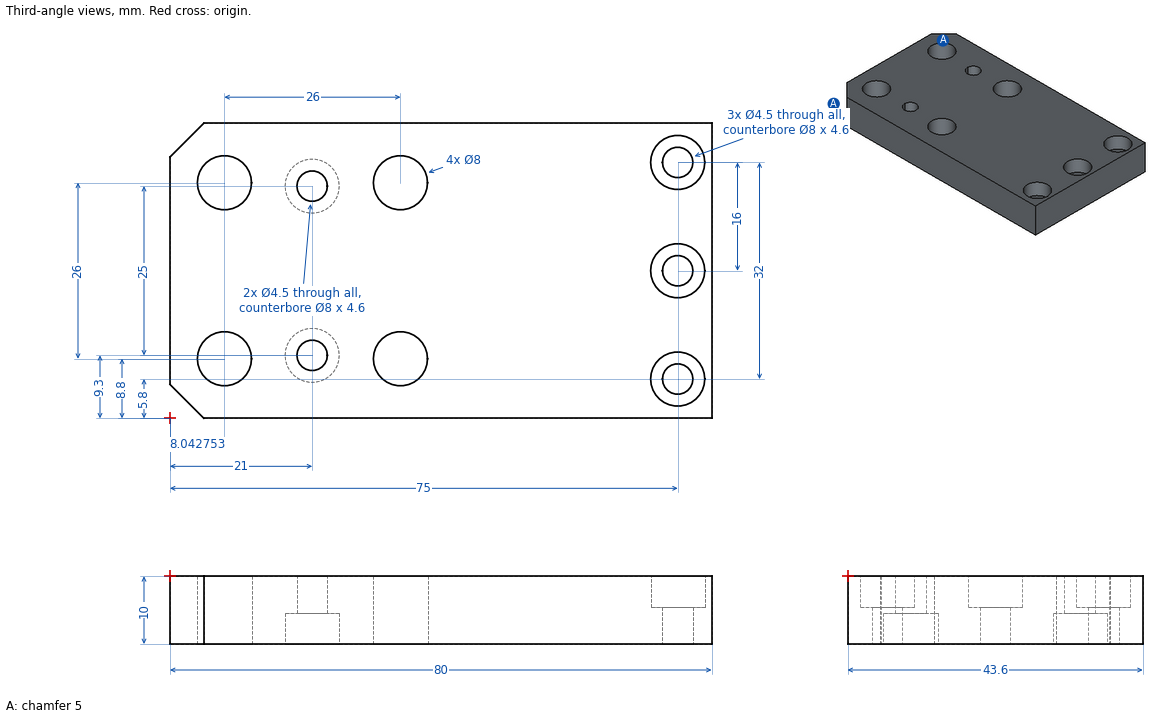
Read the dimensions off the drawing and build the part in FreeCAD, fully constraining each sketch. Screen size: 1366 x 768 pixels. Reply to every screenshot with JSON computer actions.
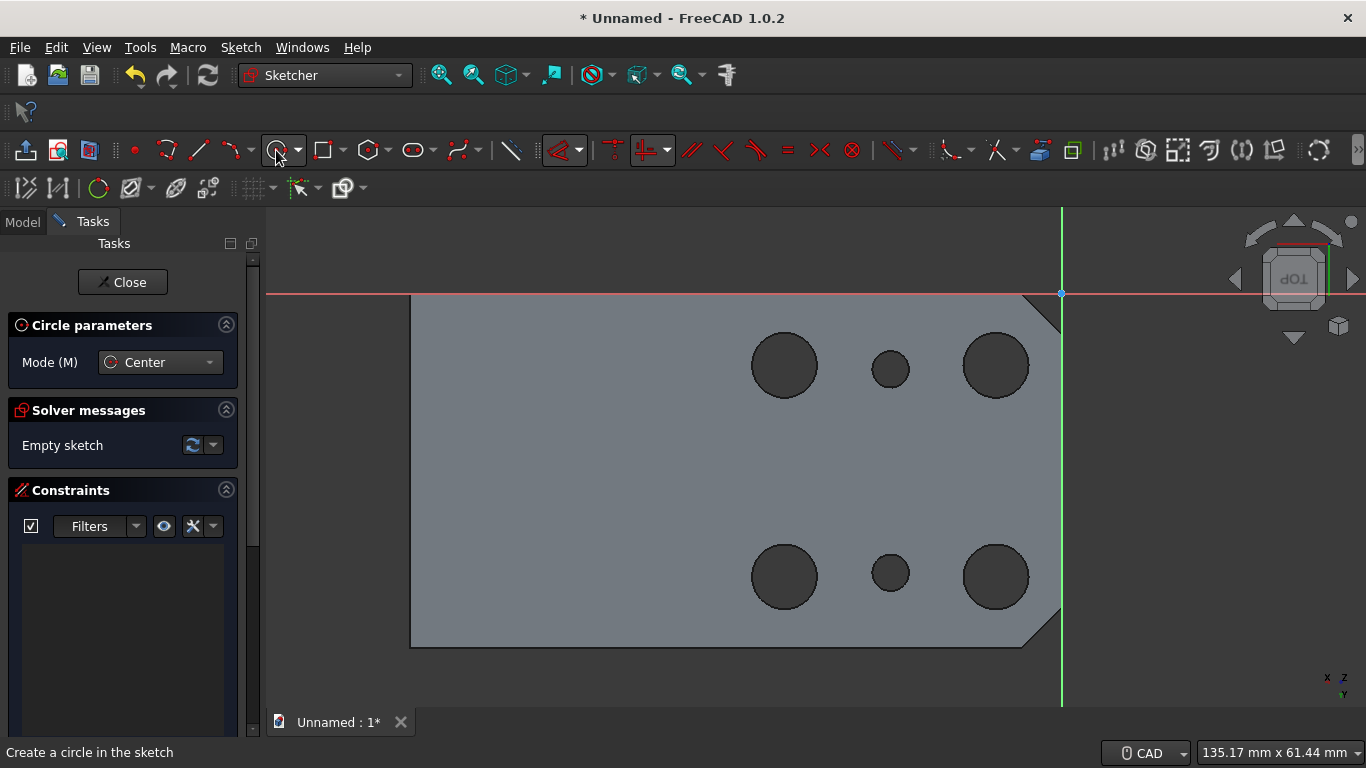
{"action": "scroll", "coordinate": [451, 601], "scroll_direction": "up", "scroll_amount": 2}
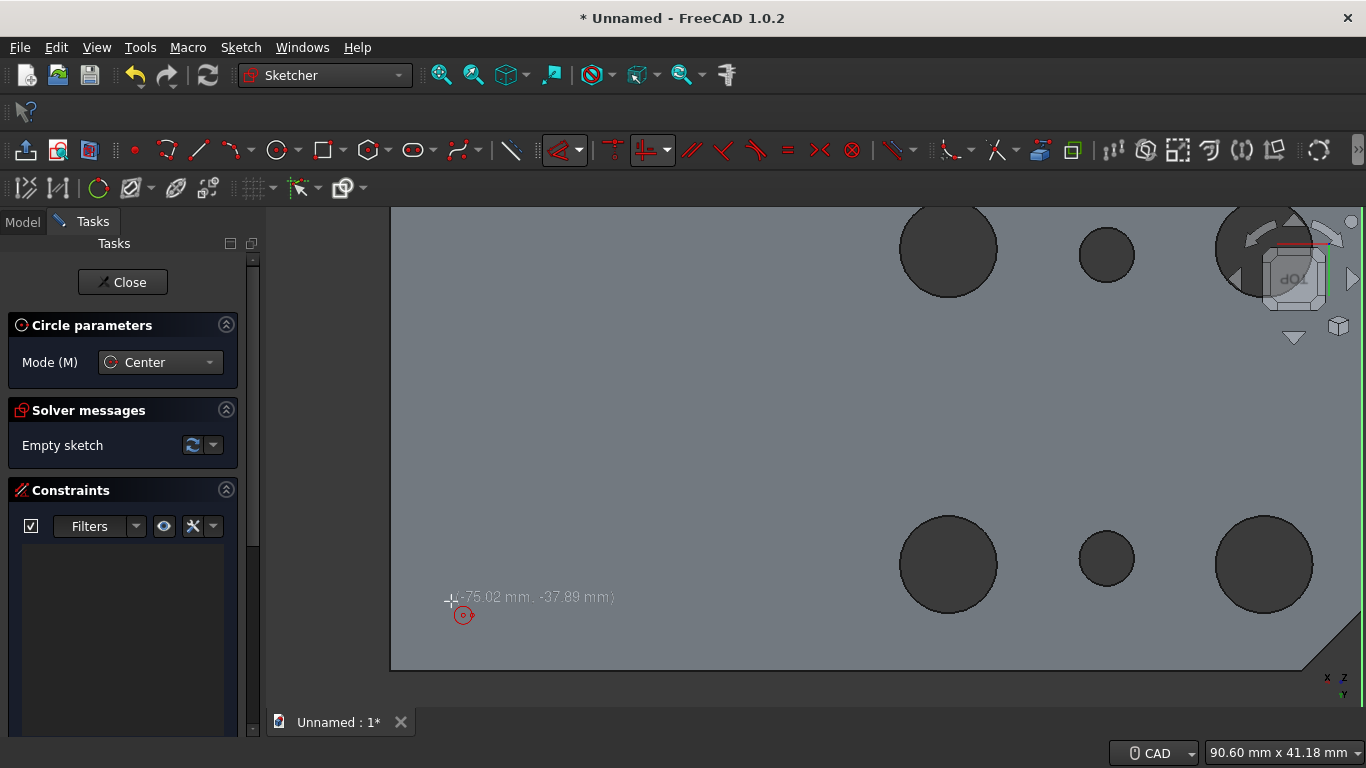
{"action": "left_click", "coordinate": [451, 601]}
{"action": "left_click", "coordinate": [470, 582]}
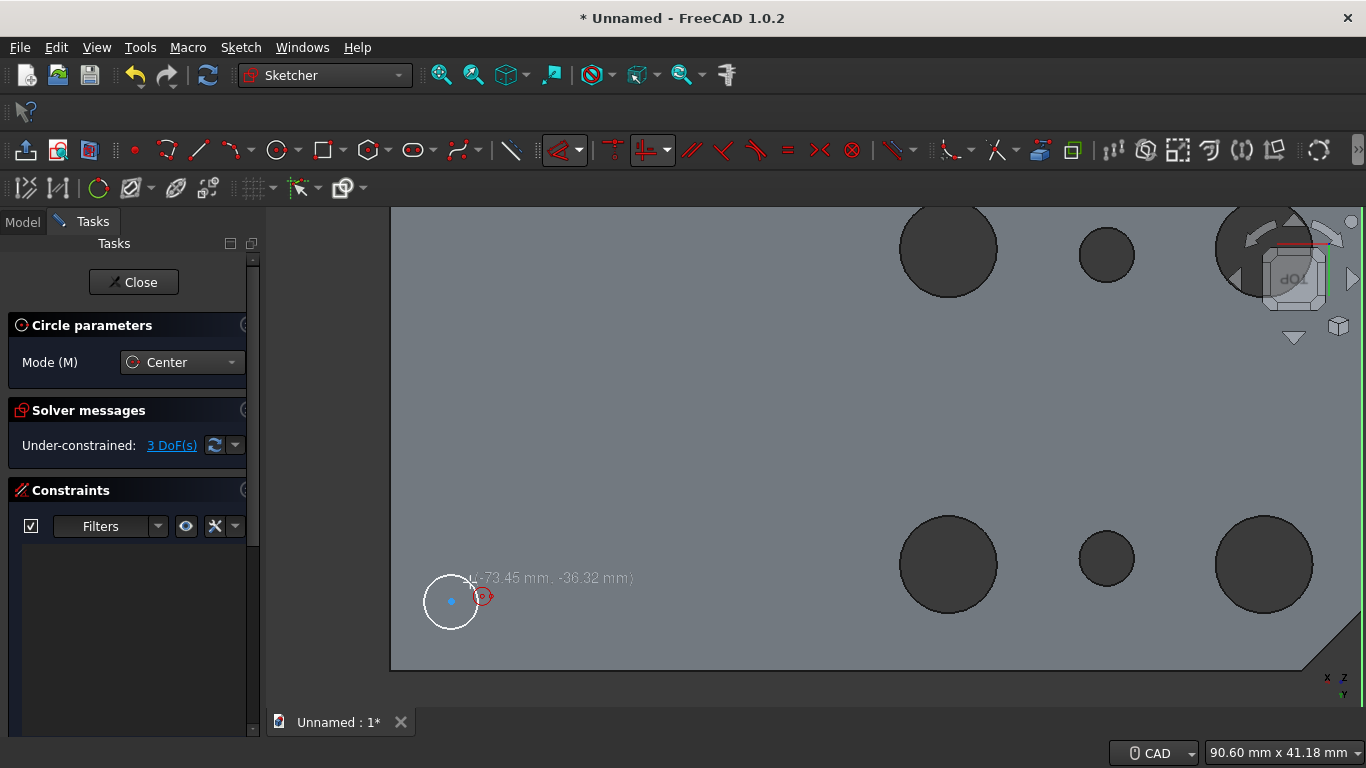
{"action": "scroll", "coordinate": [452, 603], "scroll_direction": "down", "scroll_amount": 2}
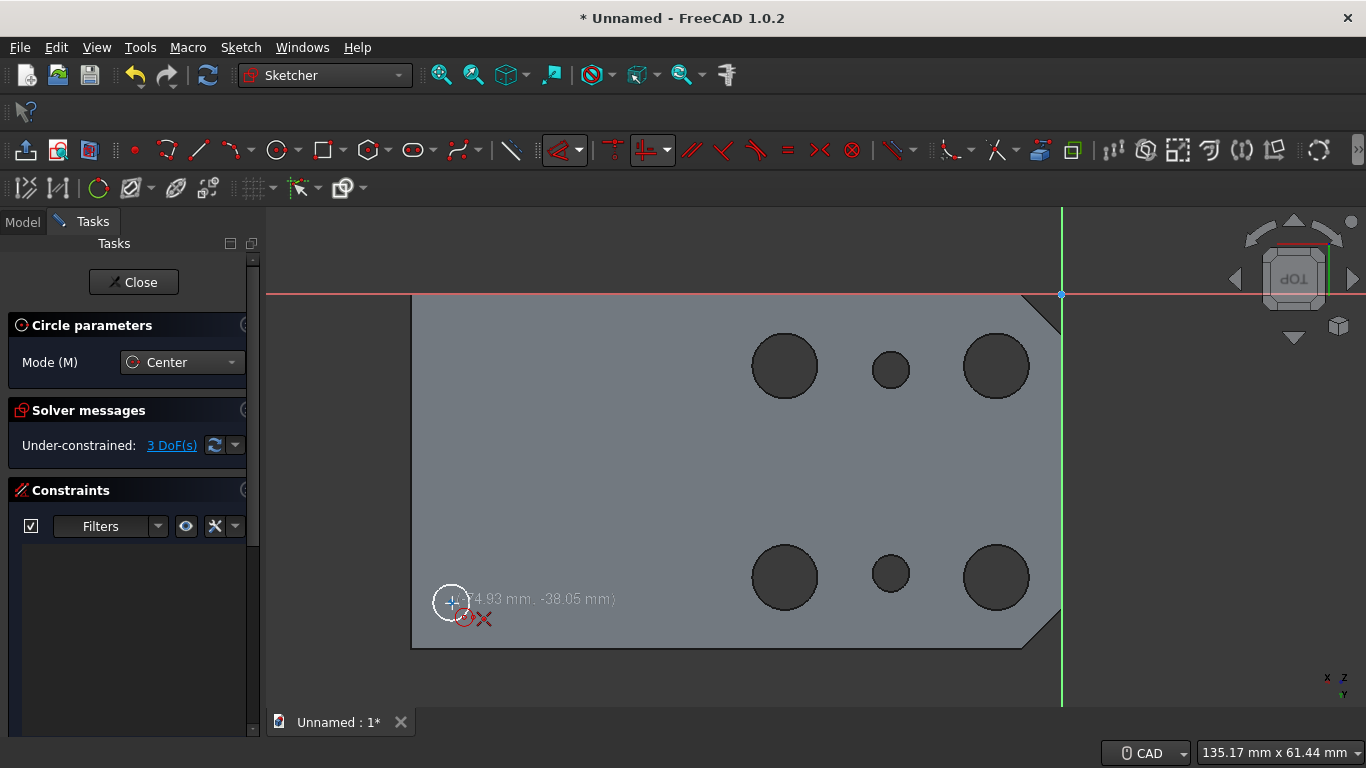
{"action": "scroll", "coordinate": [452, 341], "scroll_direction": "up", "scroll_amount": 2}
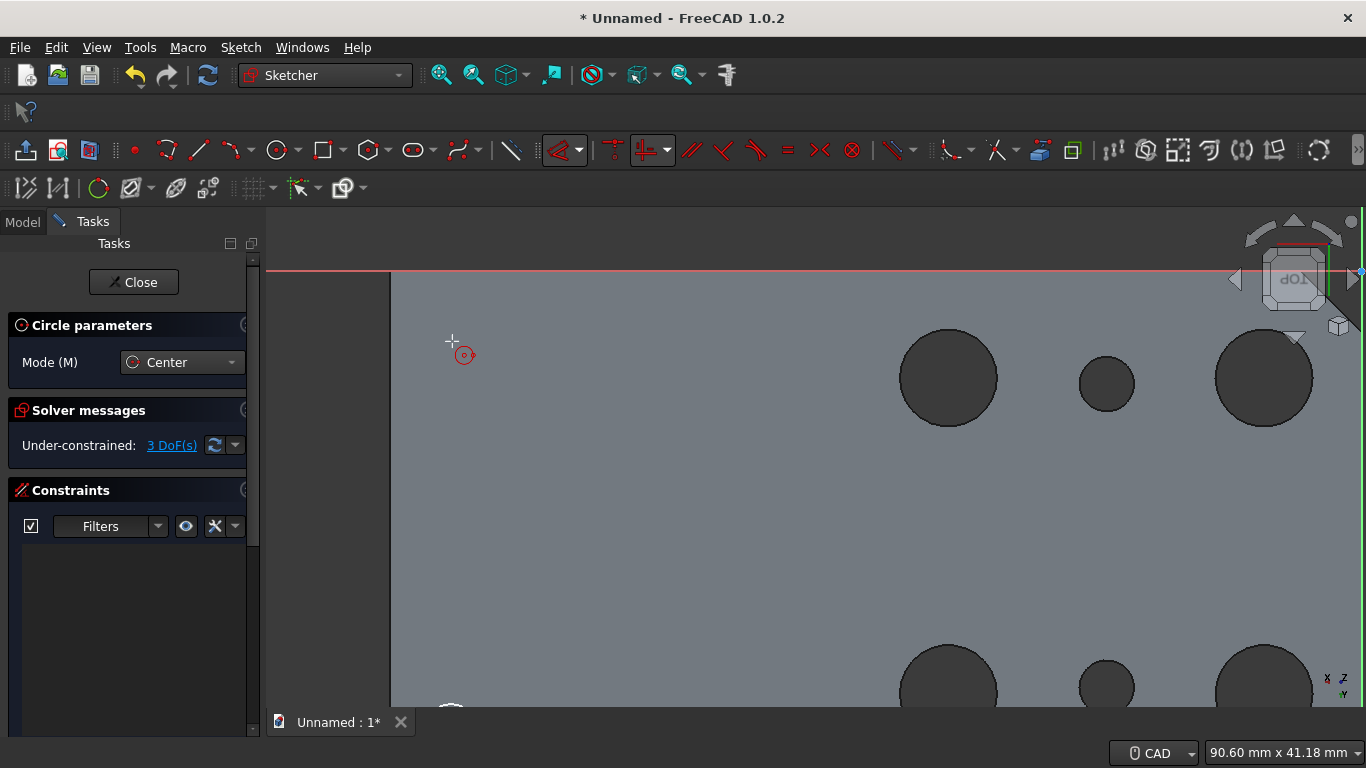
{"action": "left_click", "coordinate": [451, 342]}
{"action": "left_click", "coordinate": [470, 322]}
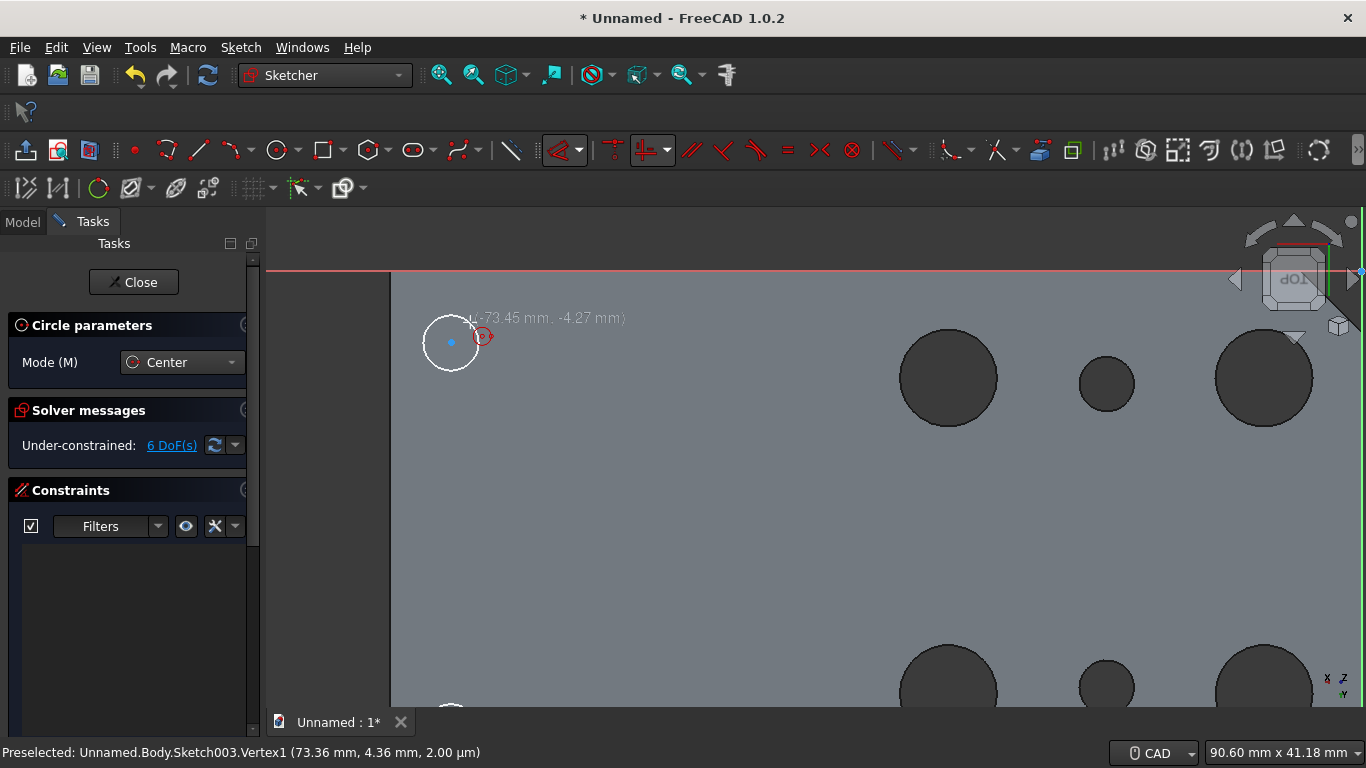
{"action": "left_click", "coordinate": [451, 536]}
{"action": "left_click", "coordinate": [470, 517]}
{"action": "key", "text": "Escape"}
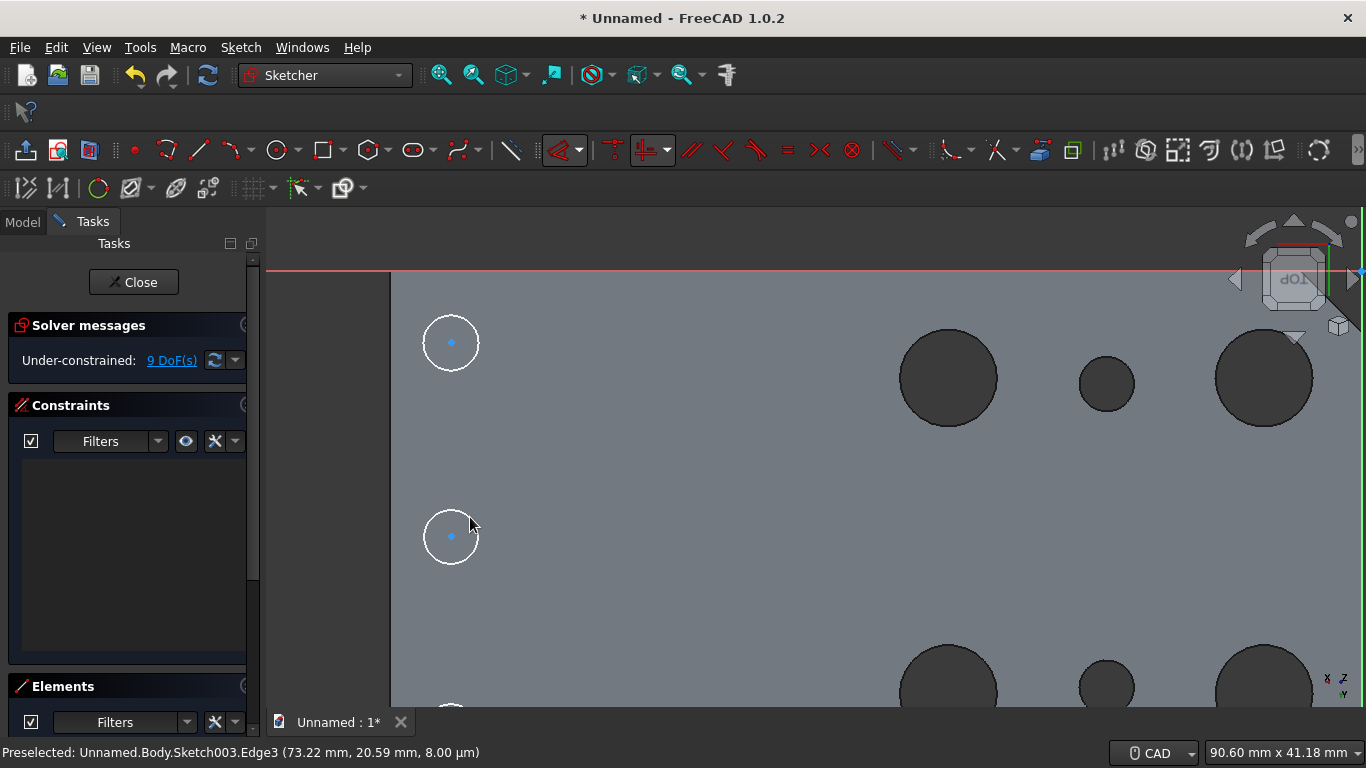
{"action": "scroll", "coordinate": [452, 340], "scroll_direction": "down", "scroll_amount": 2}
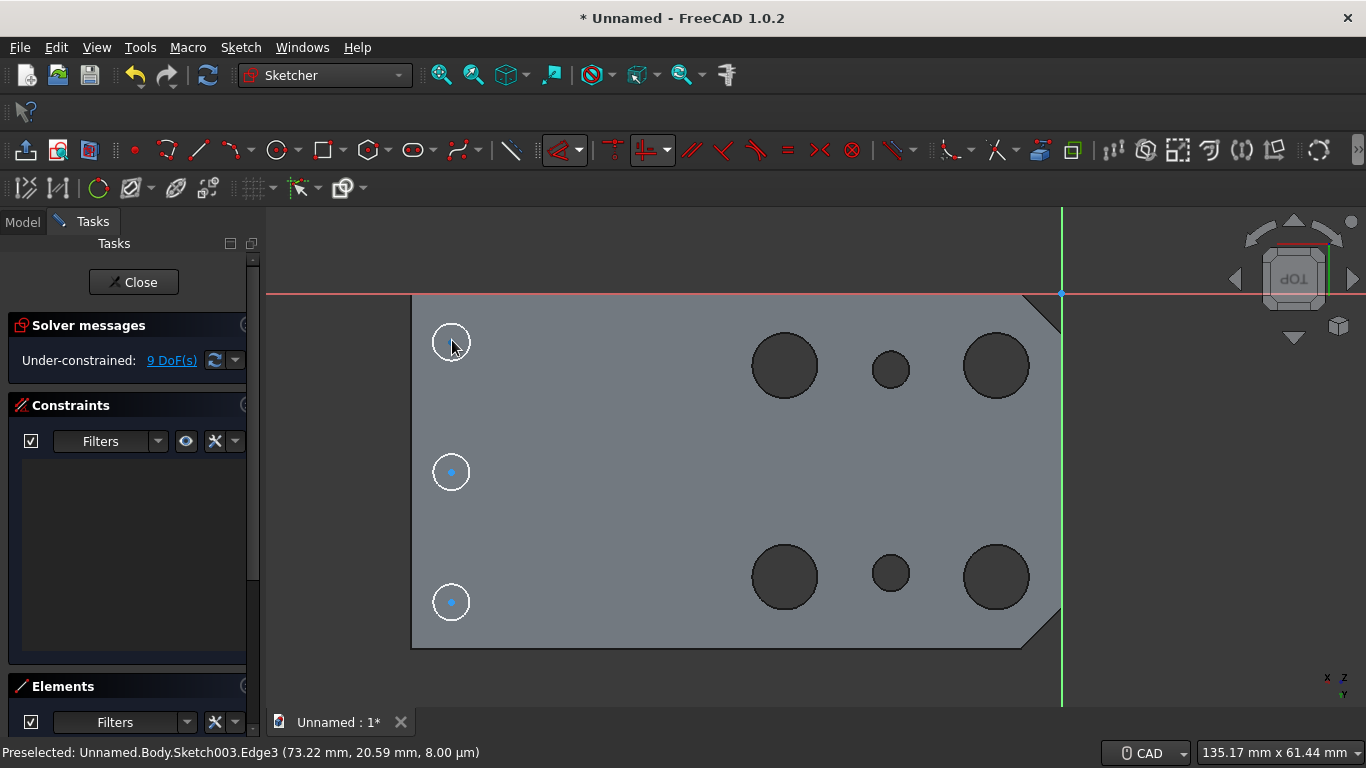
{"action": "left_click", "coordinate": [464, 589]}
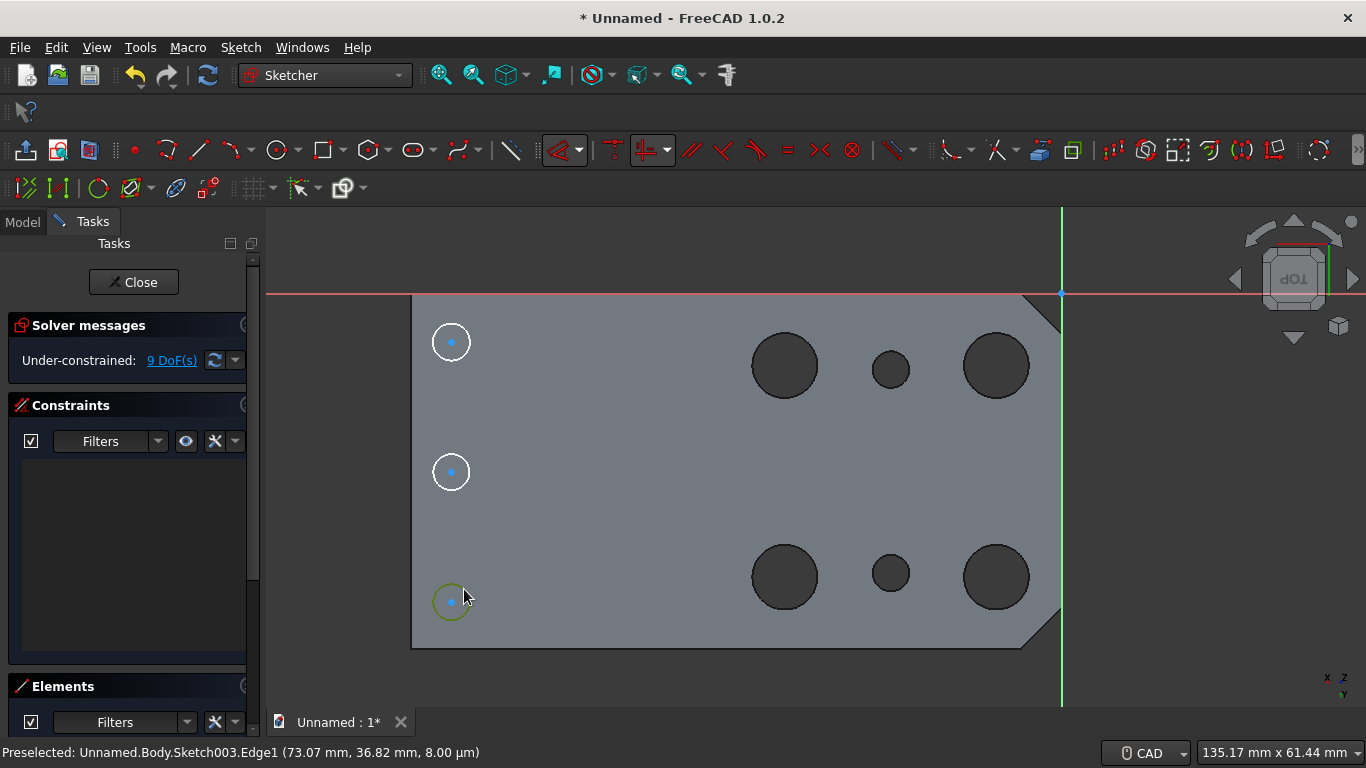
{"action": "left_click", "coordinate": [464, 329]}